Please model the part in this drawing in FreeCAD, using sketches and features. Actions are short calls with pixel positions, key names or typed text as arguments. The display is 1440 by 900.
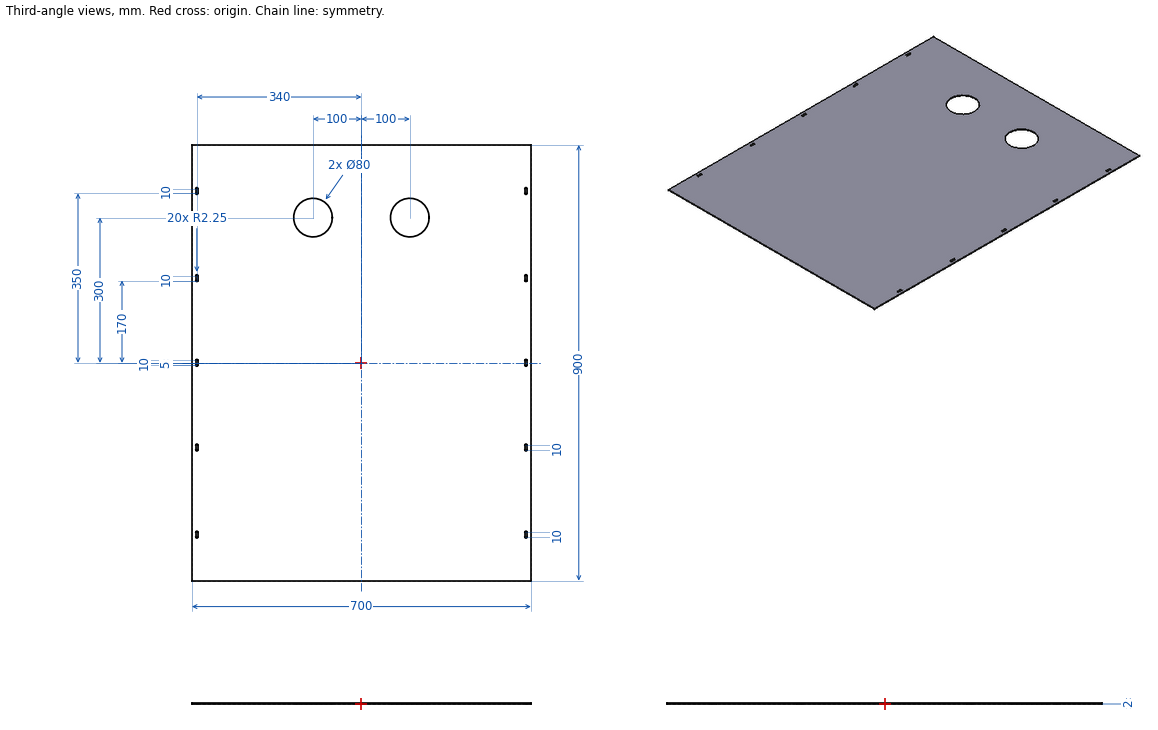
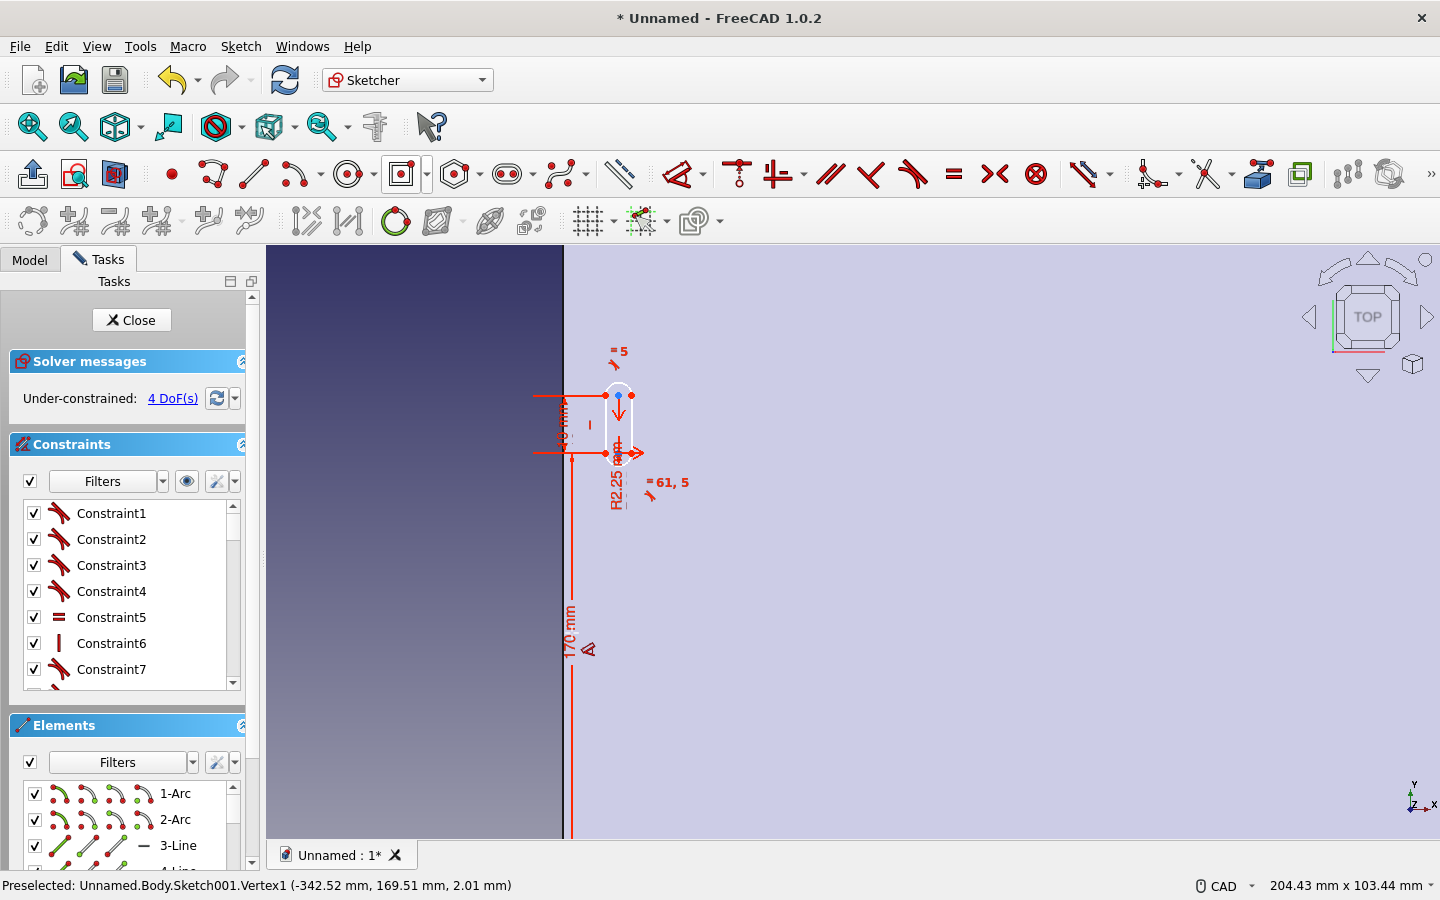
scroll(606, 453, down, 12)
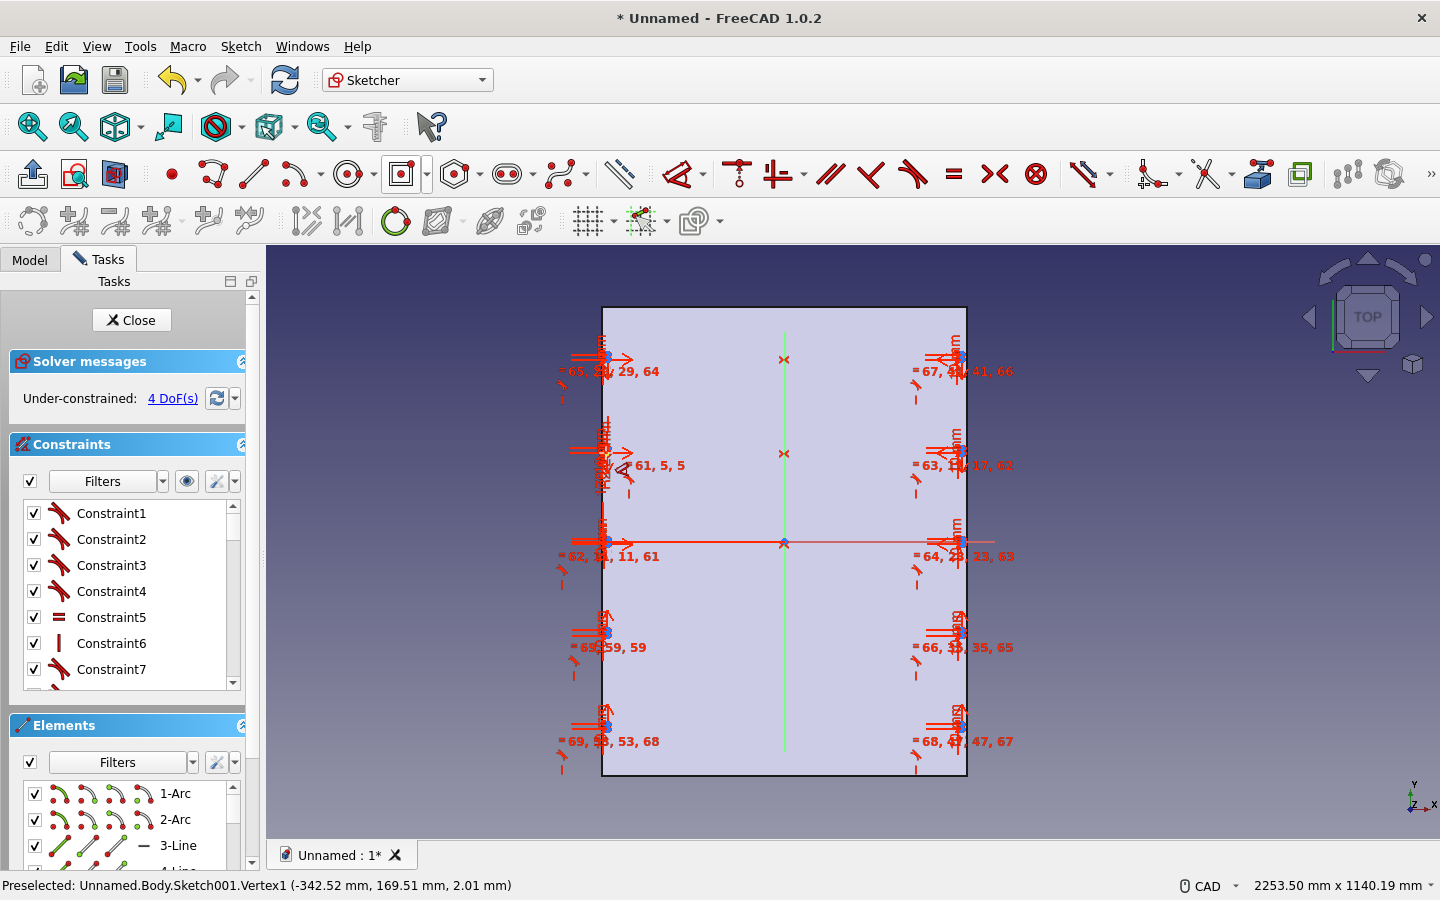
scroll(606, 360, up, 12)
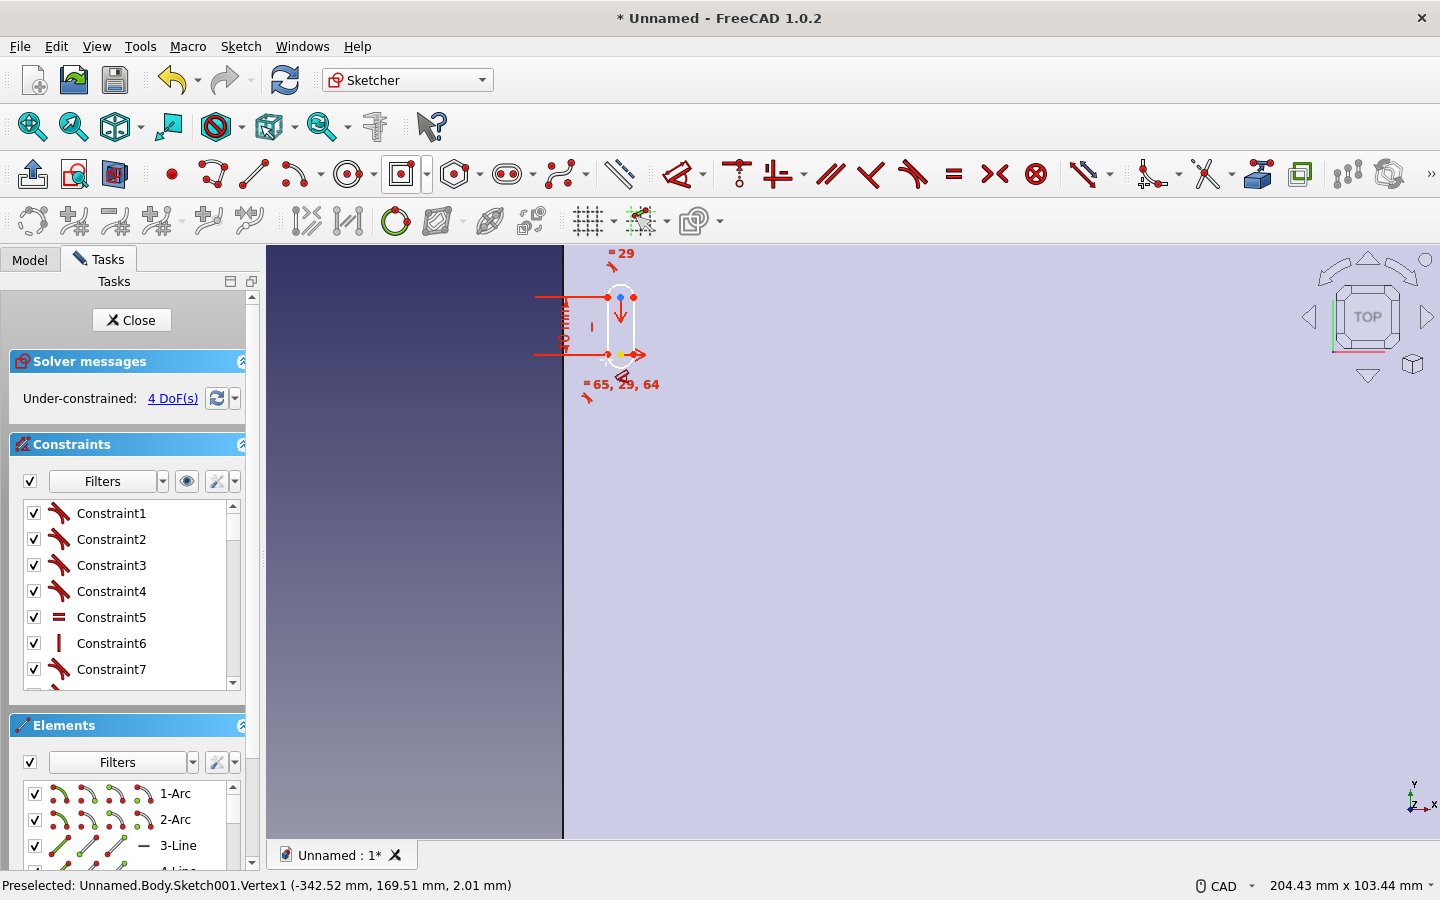
click(608, 355)
click(574, 583)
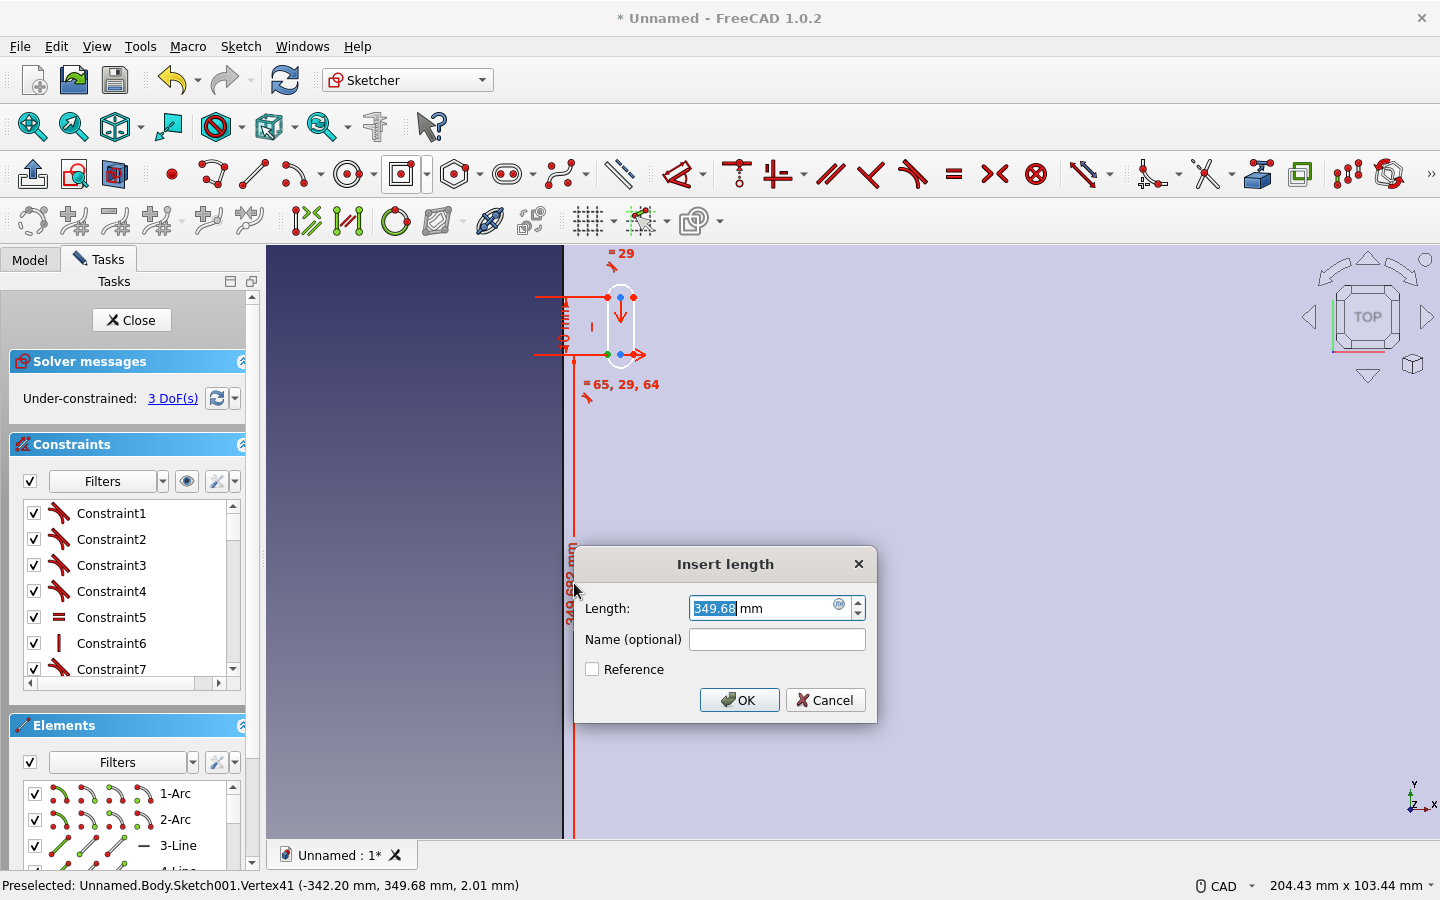
text(350)
key(Return)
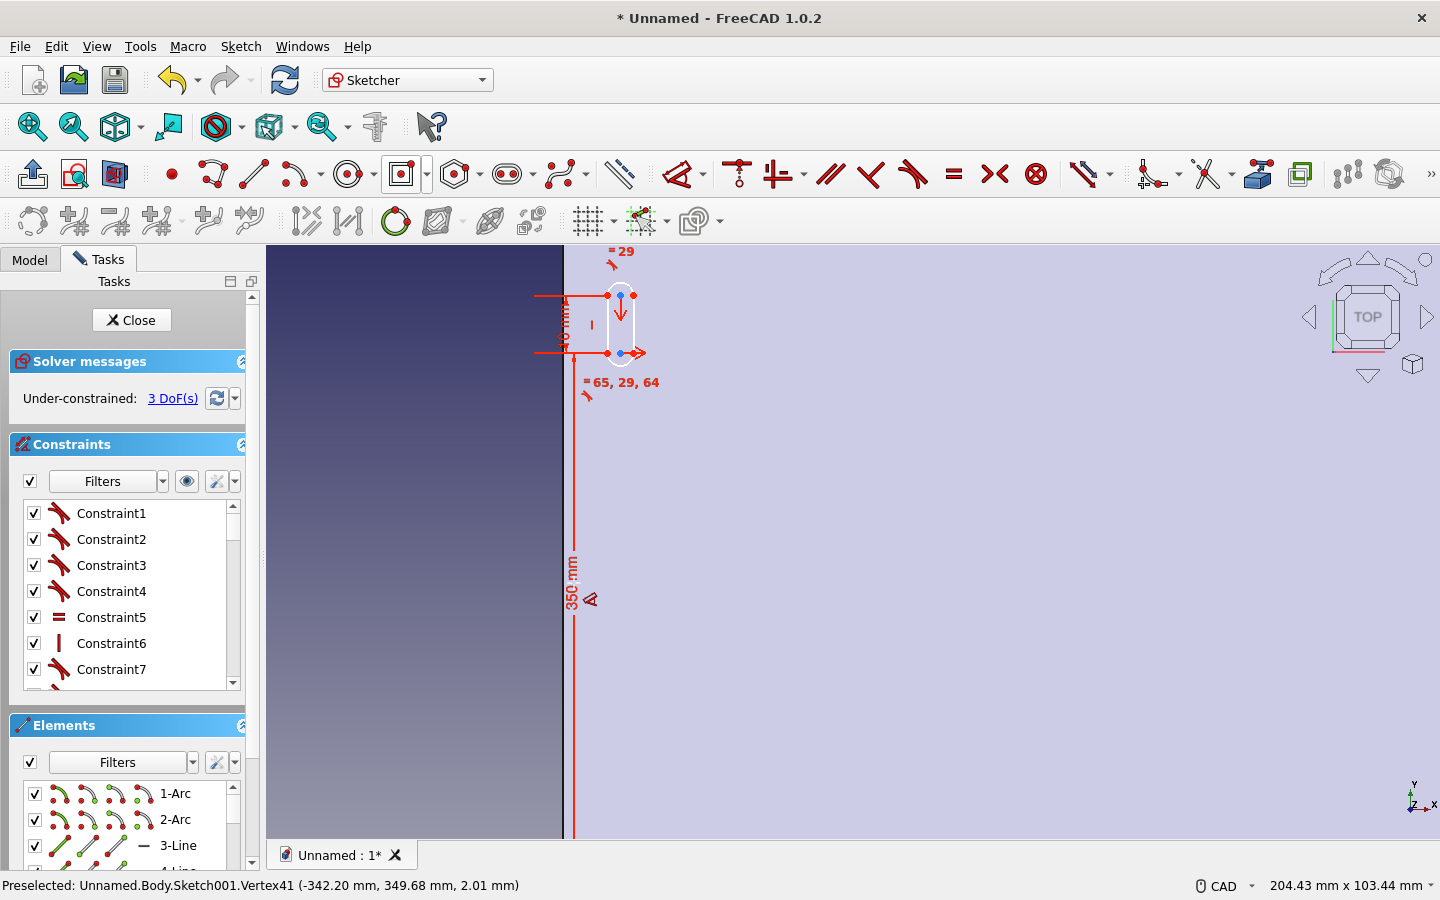
scroll(606, 360, down, 12)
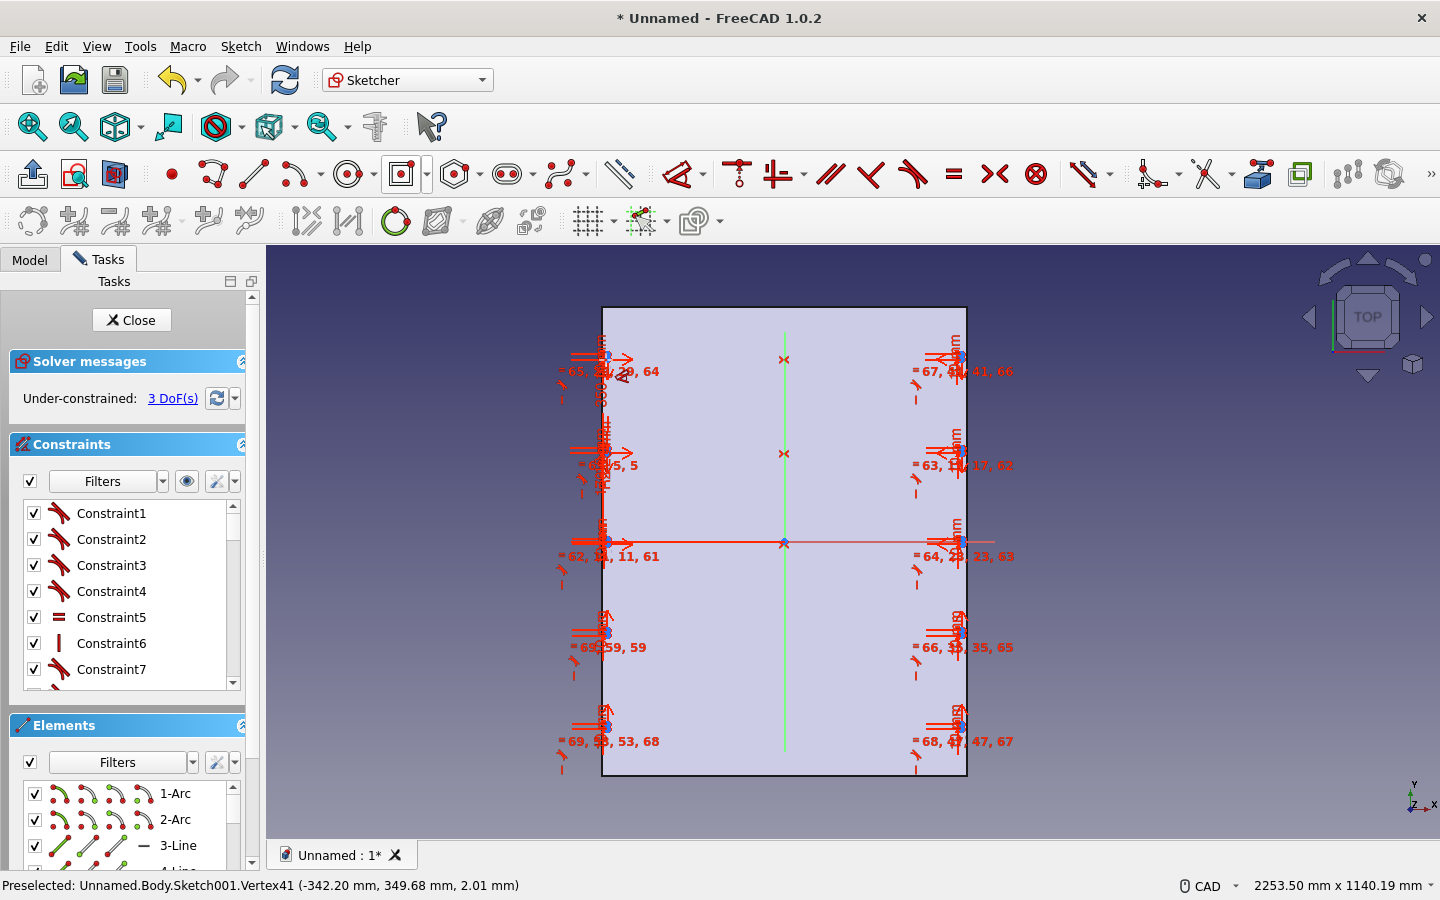
scroll(607, 453, up, 12)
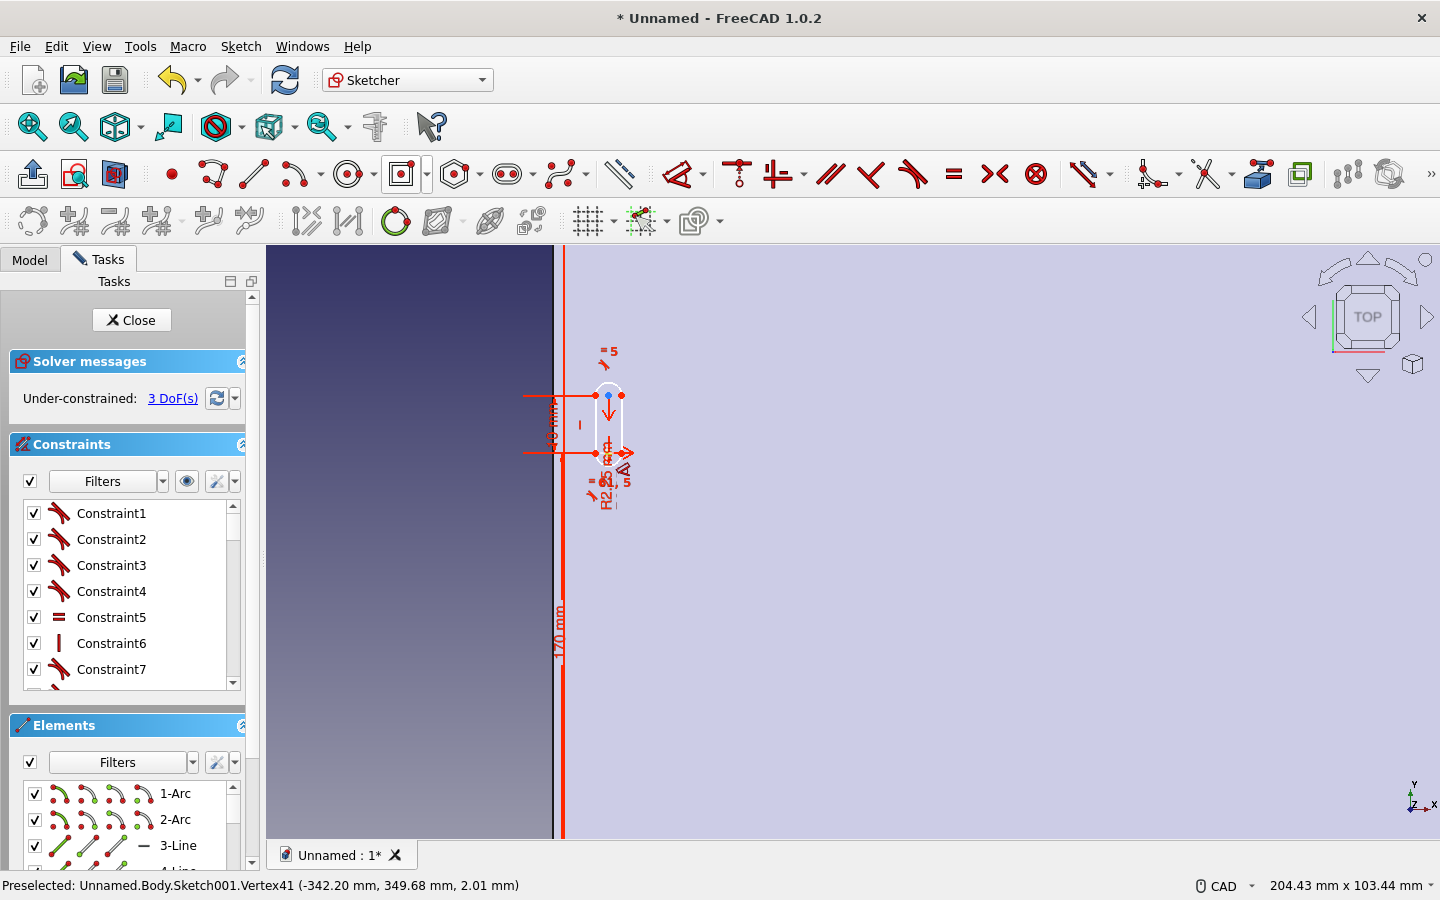
click(609, 453)
click(942, 419)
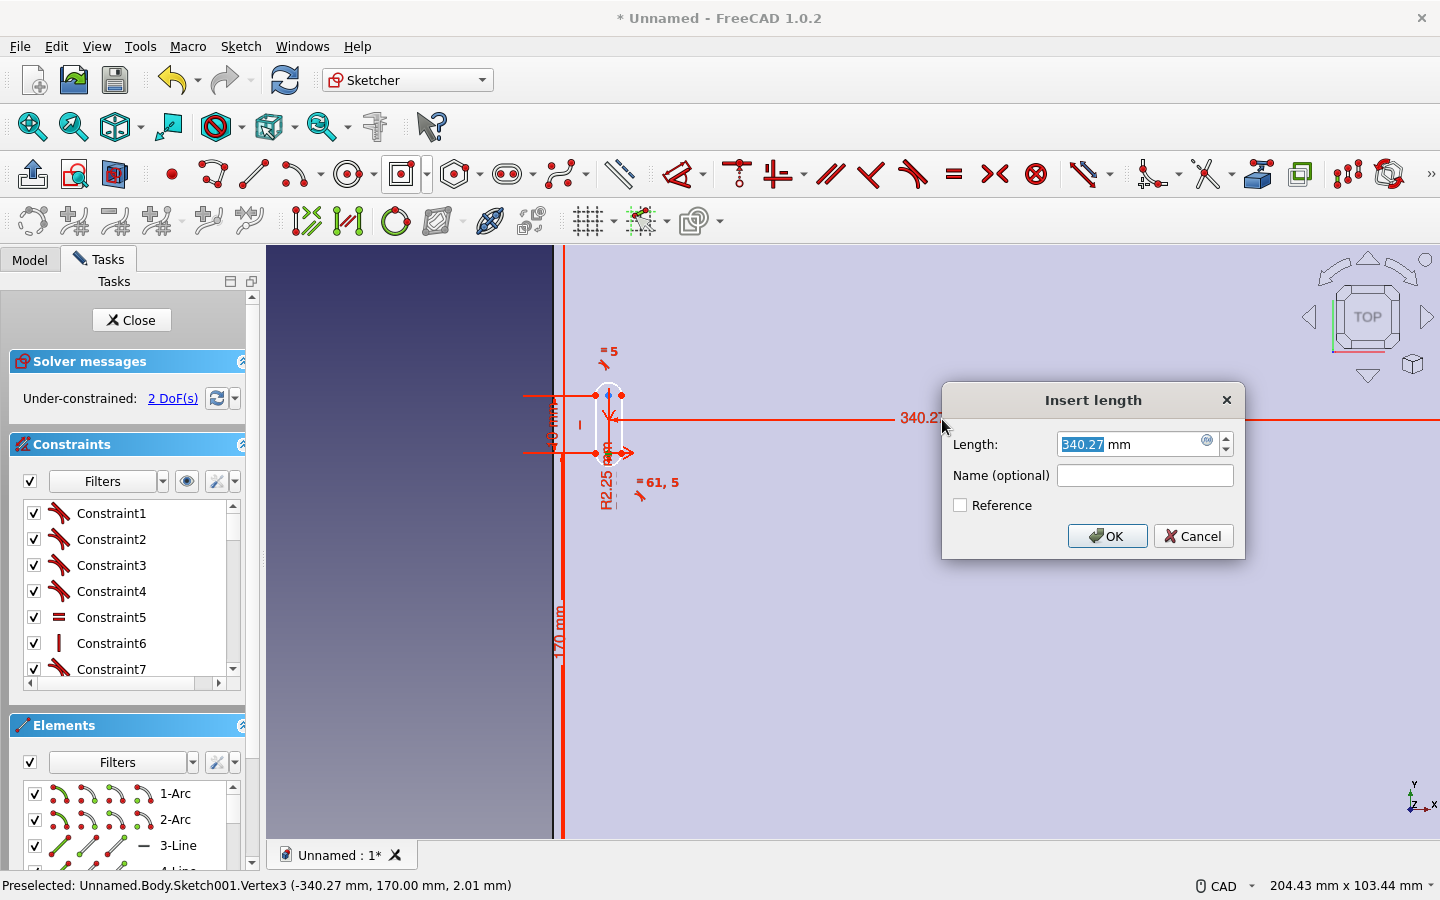
text(340)
key(Return)